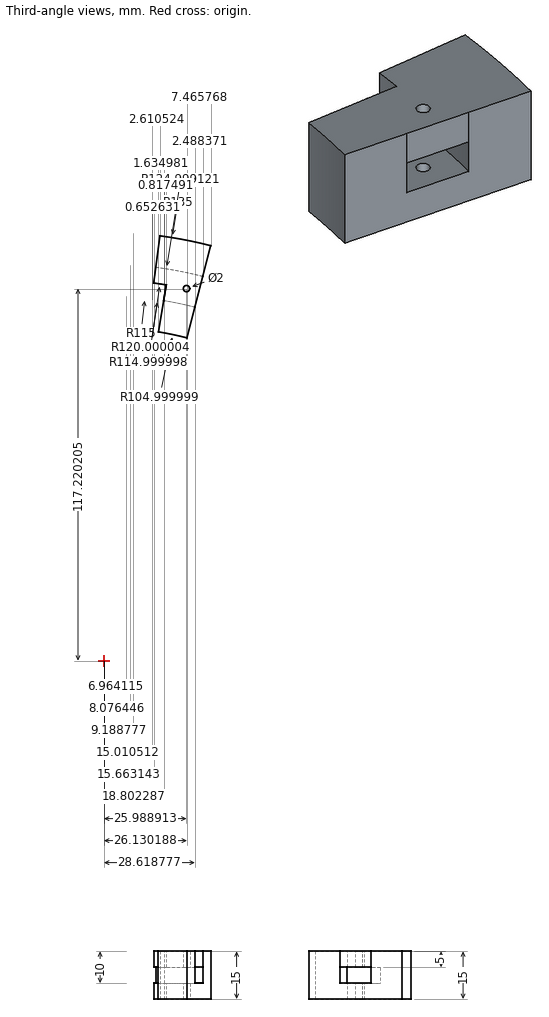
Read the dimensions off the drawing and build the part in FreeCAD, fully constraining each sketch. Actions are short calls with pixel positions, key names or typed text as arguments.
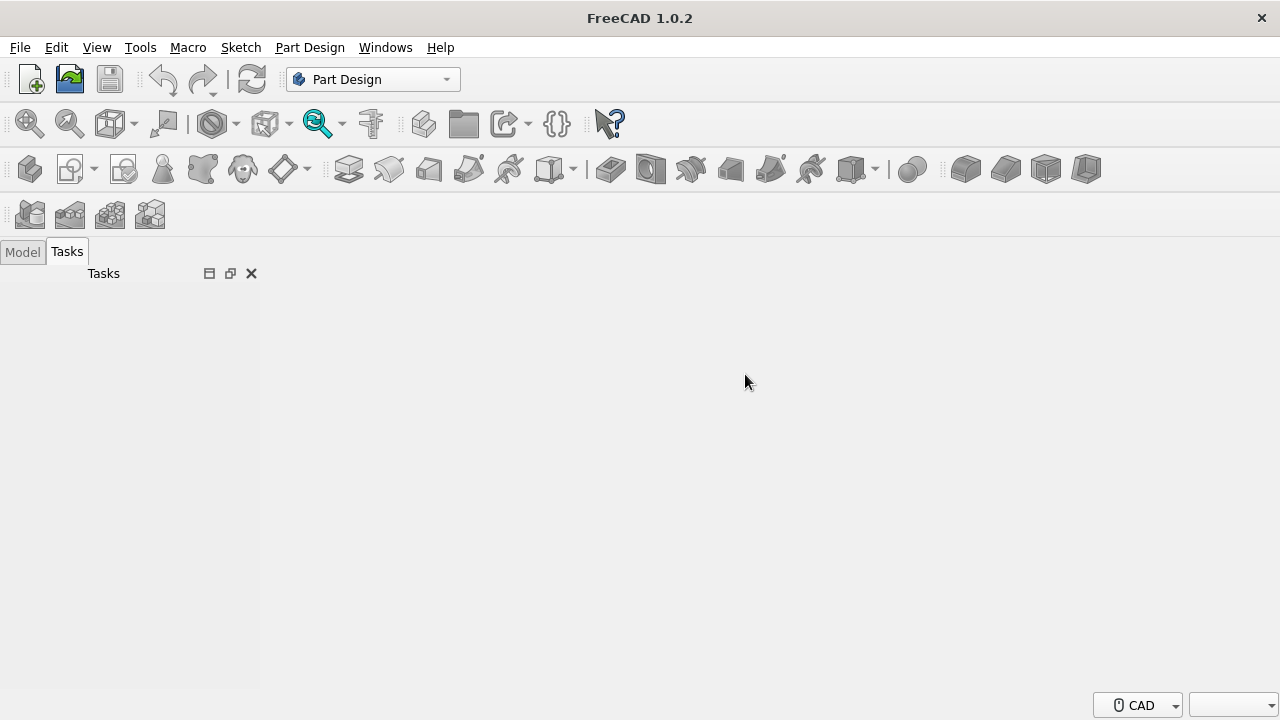
click(30, 80)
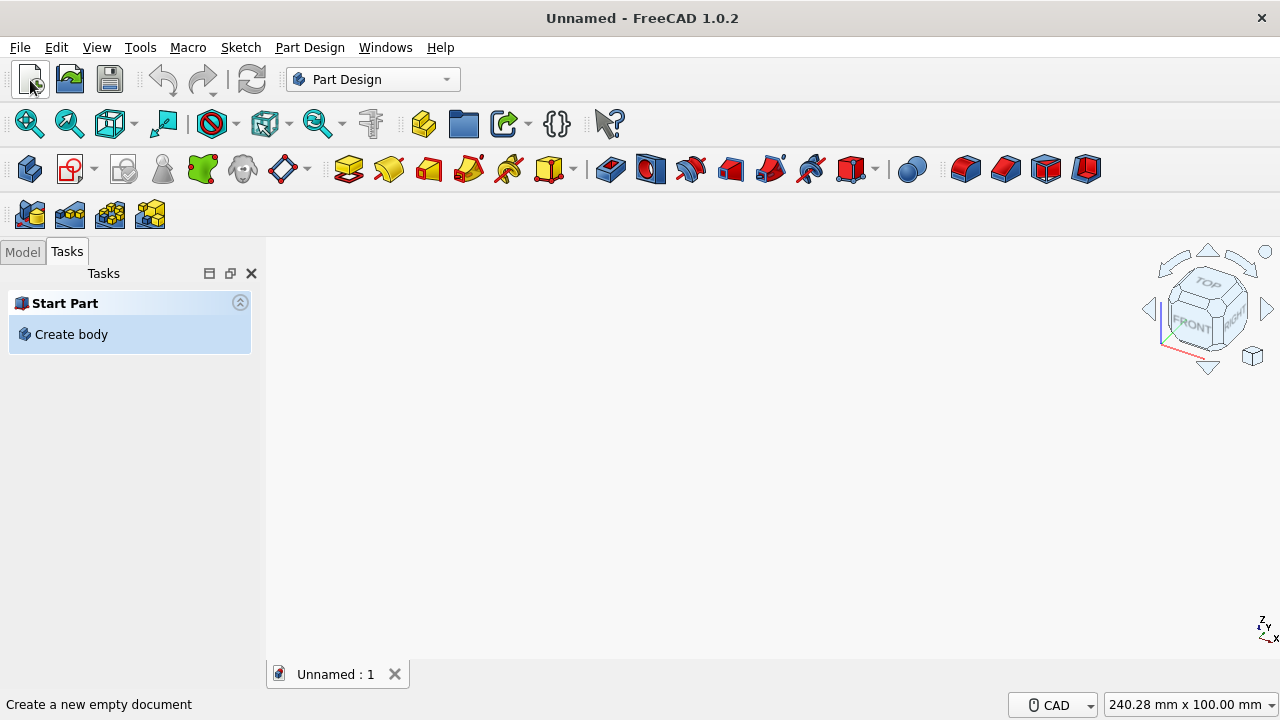
click(70, 170)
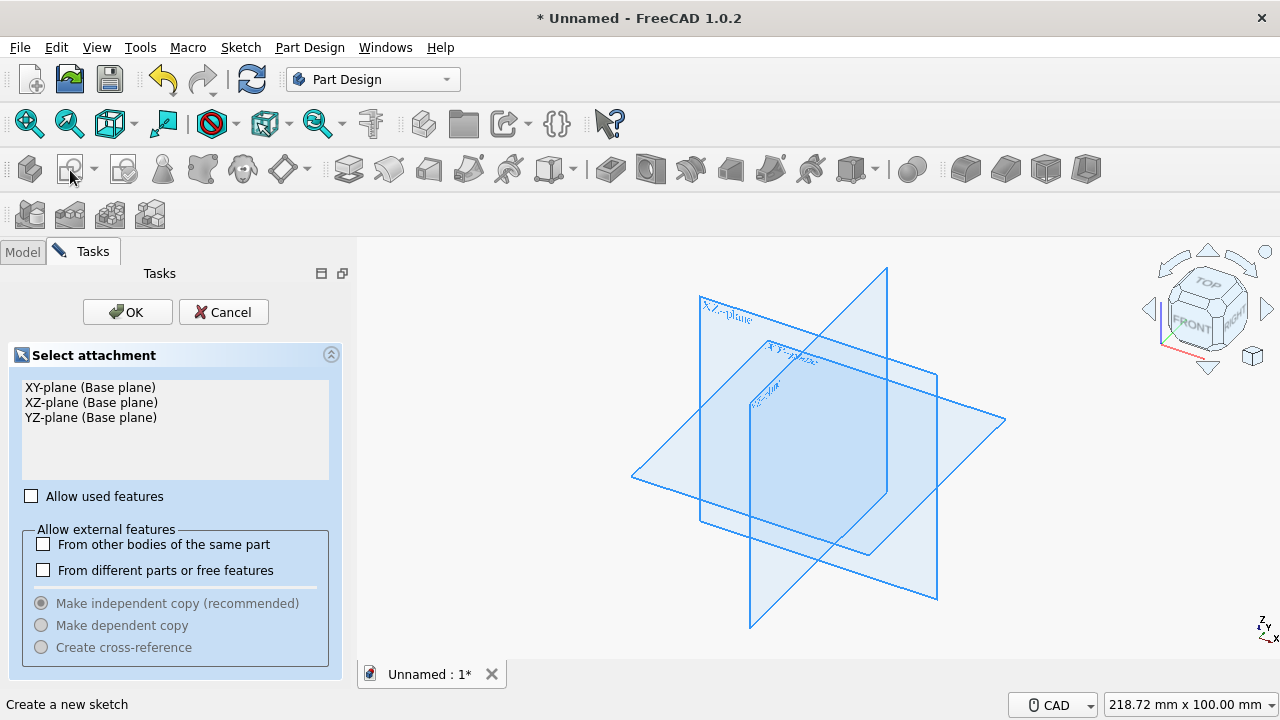
click(82, 388)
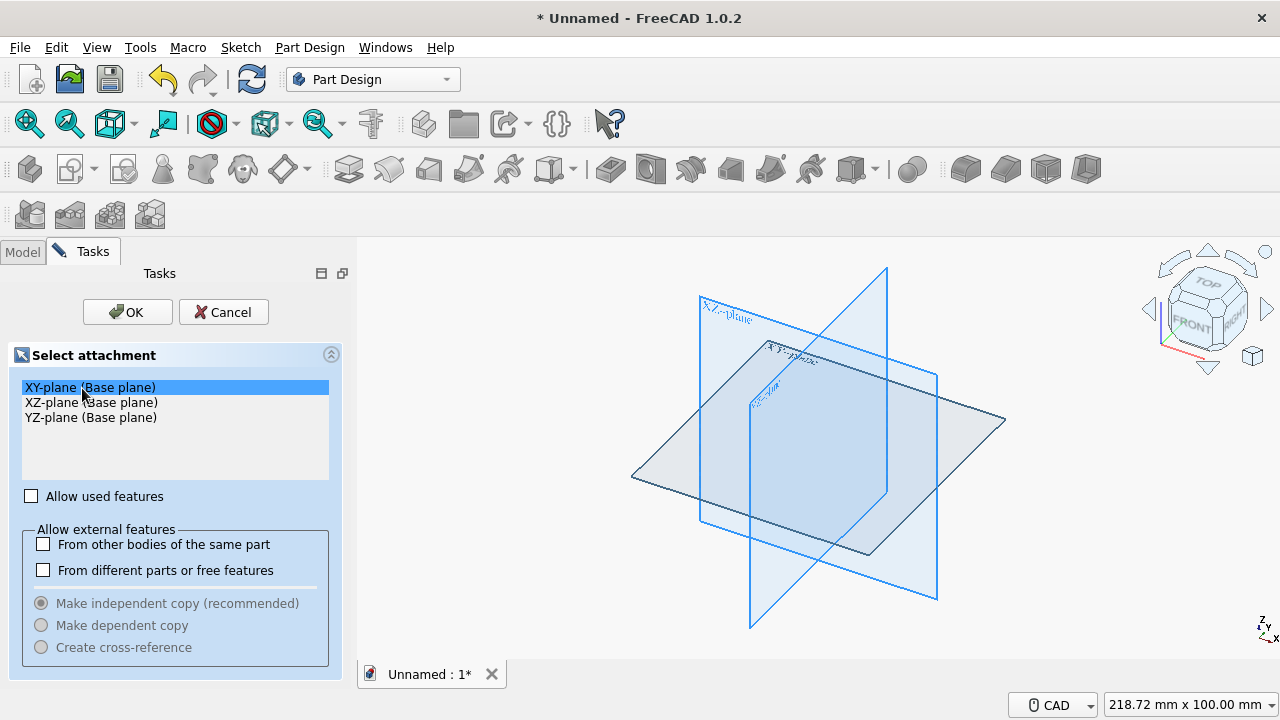
click(128, 312)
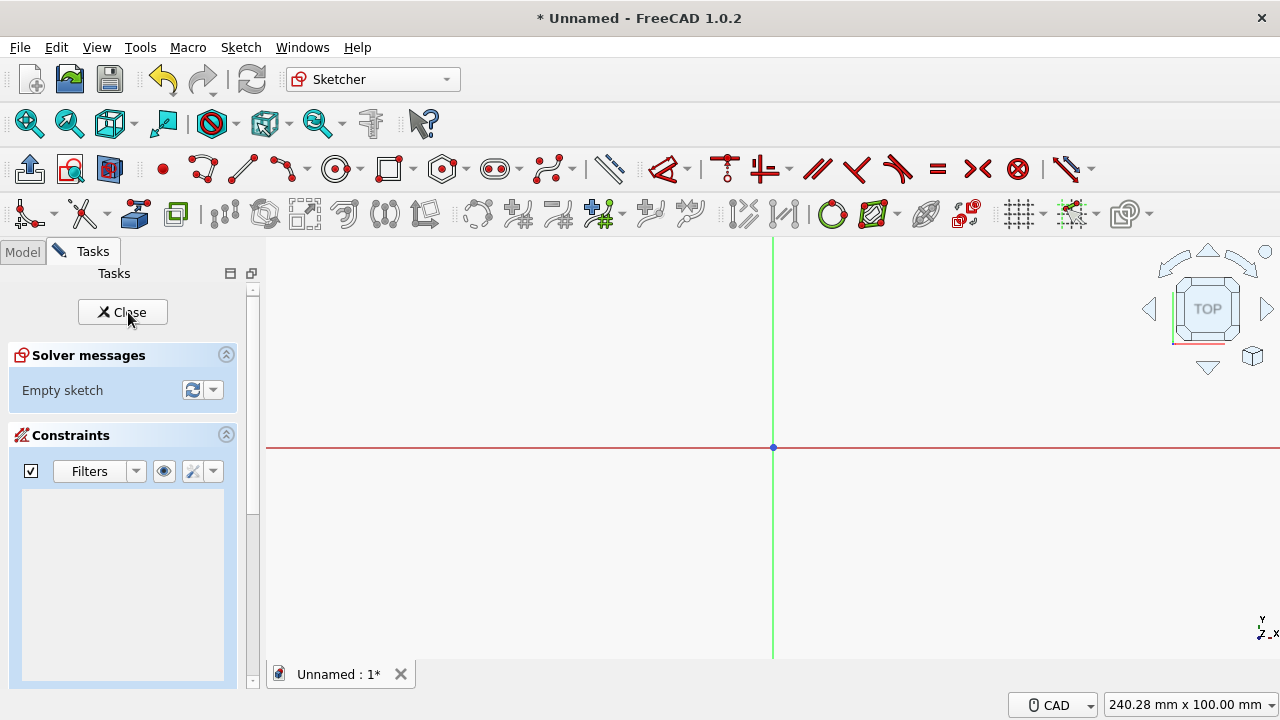
scroll(704, 448, down, 5)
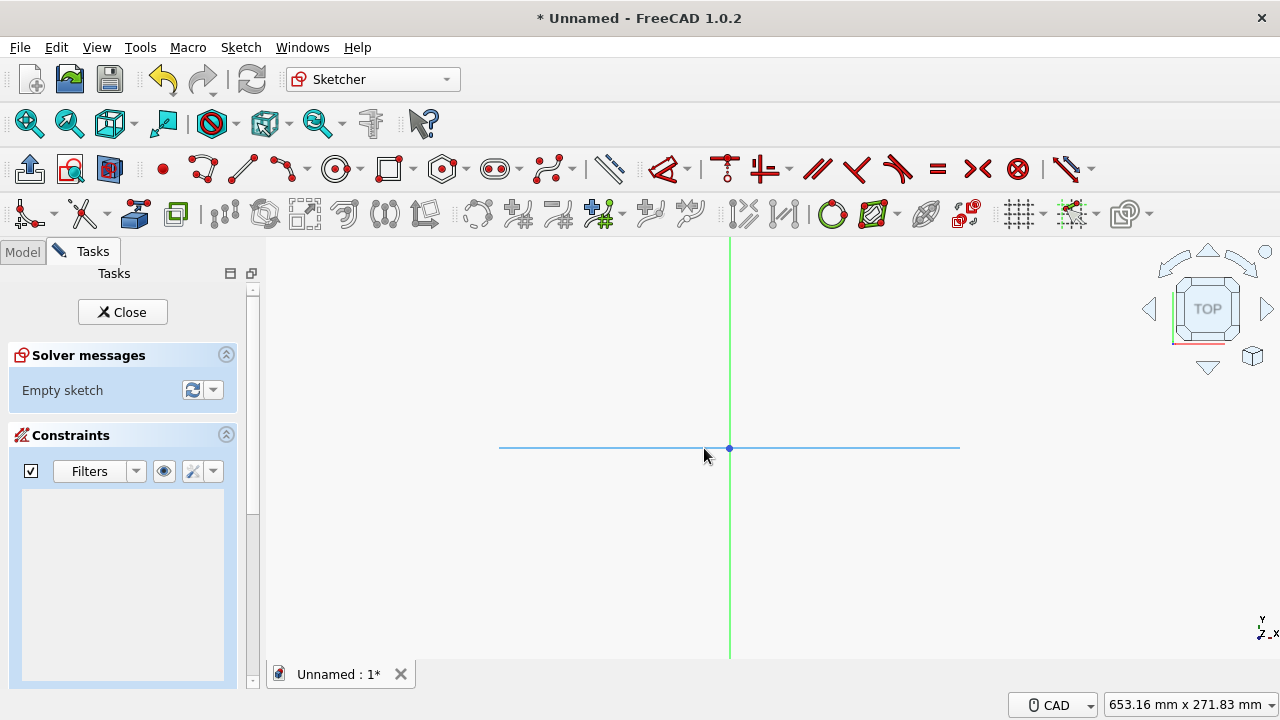
scroll(704, 448, down, 5)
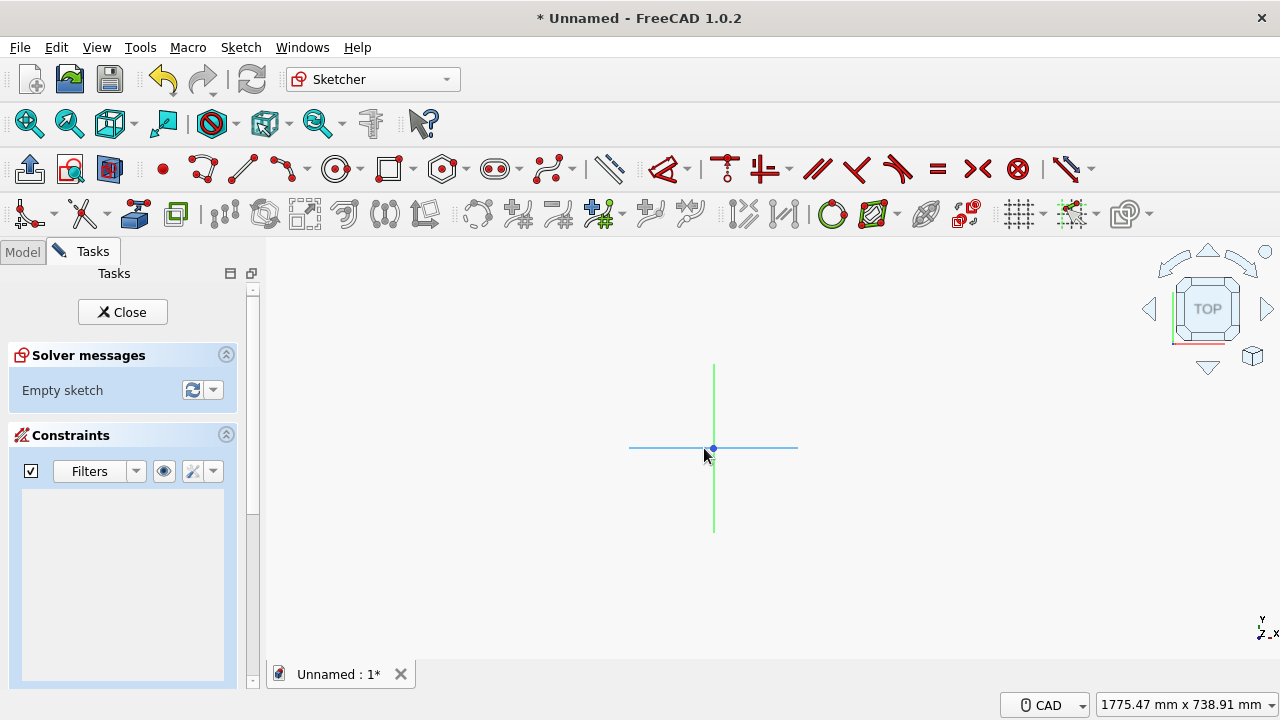
scroll(727, 376, up, 13)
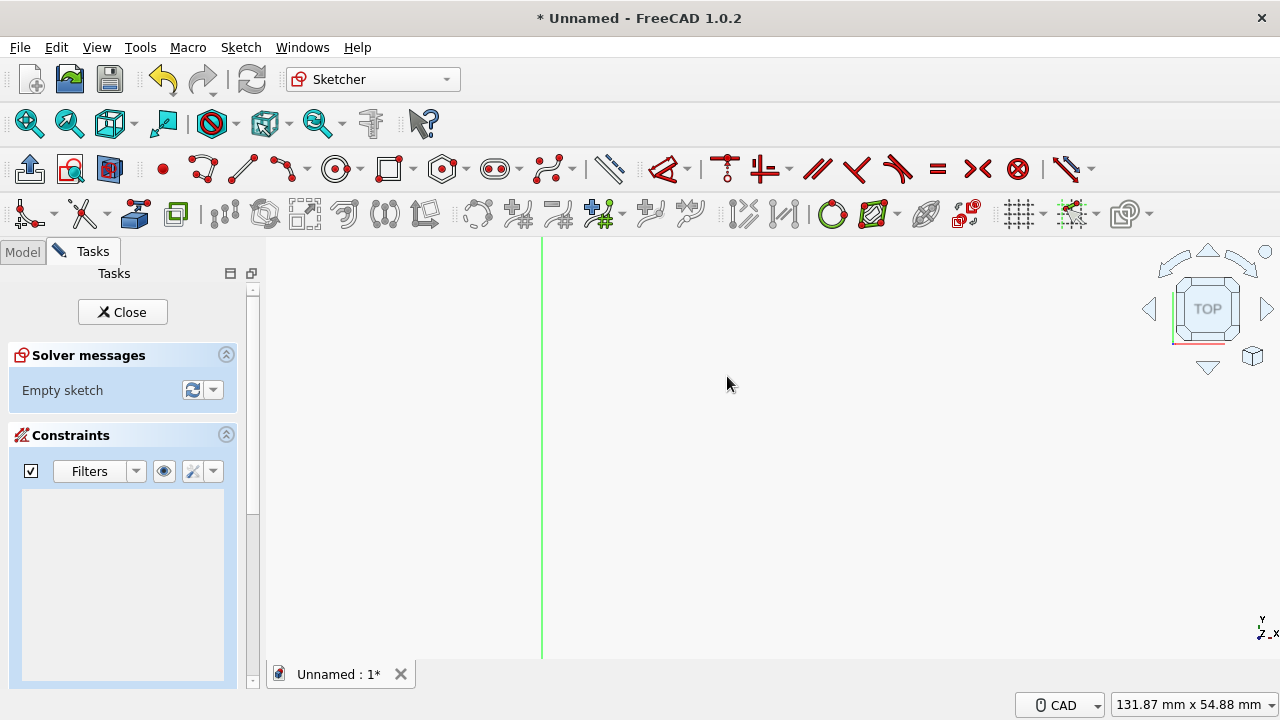
click(244, 170)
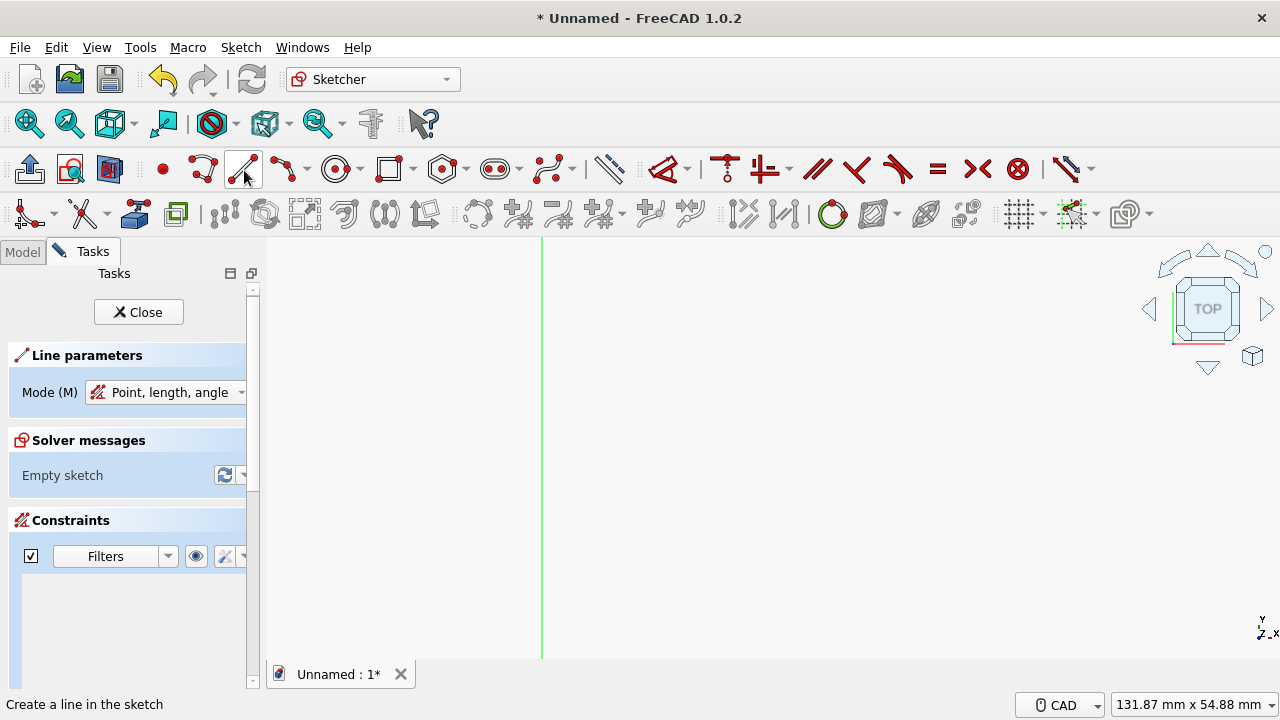
click(613, 311)
click(596, 464)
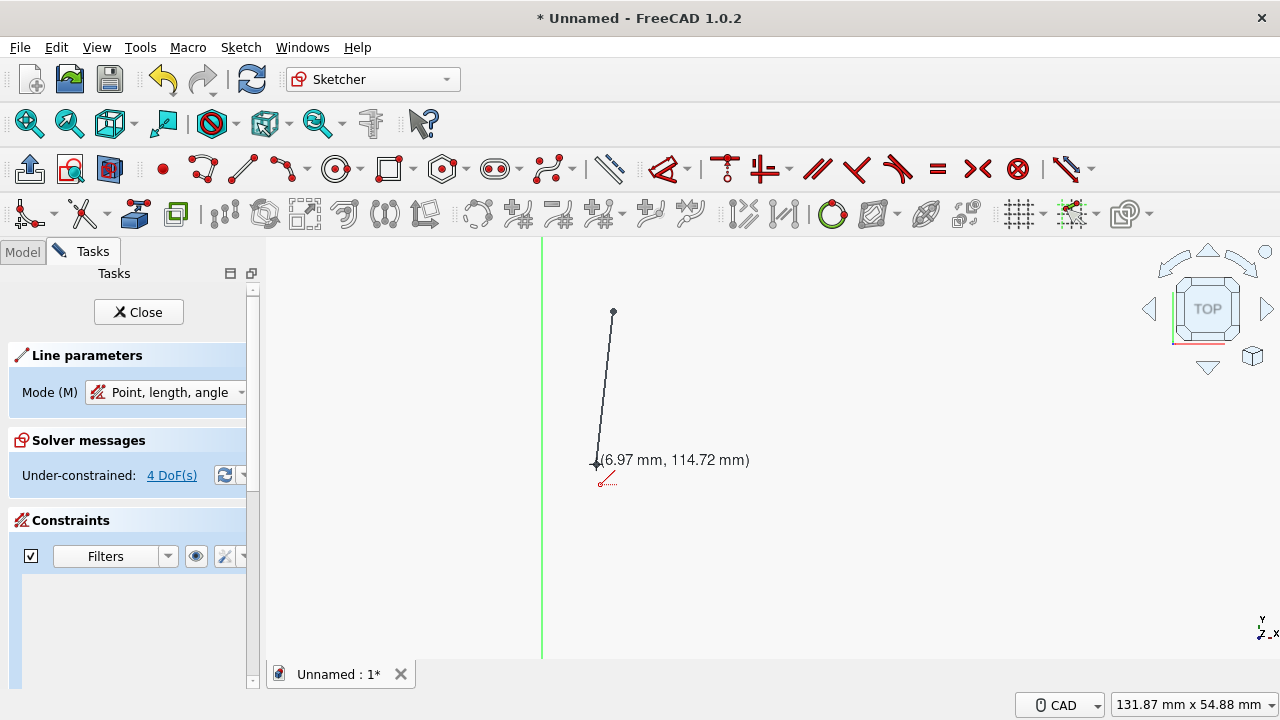
click(687, 475)
click(674, 551)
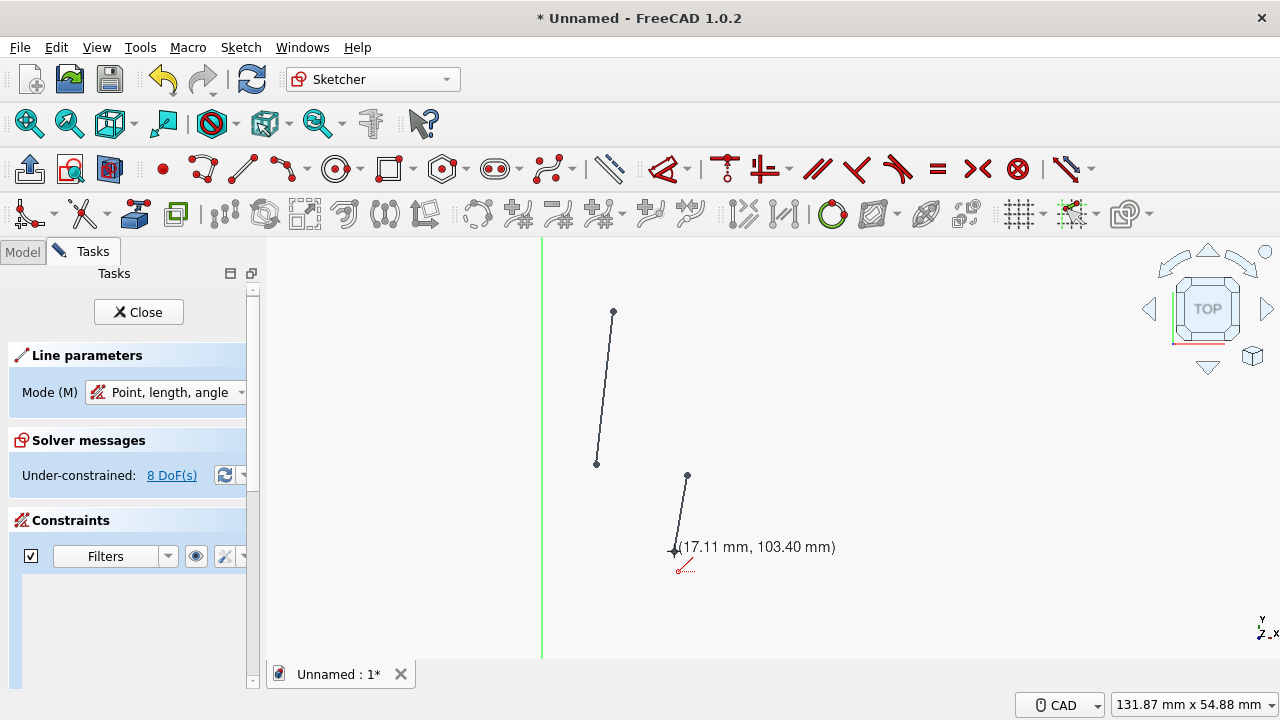
click(743, 565)
click(801, 342)